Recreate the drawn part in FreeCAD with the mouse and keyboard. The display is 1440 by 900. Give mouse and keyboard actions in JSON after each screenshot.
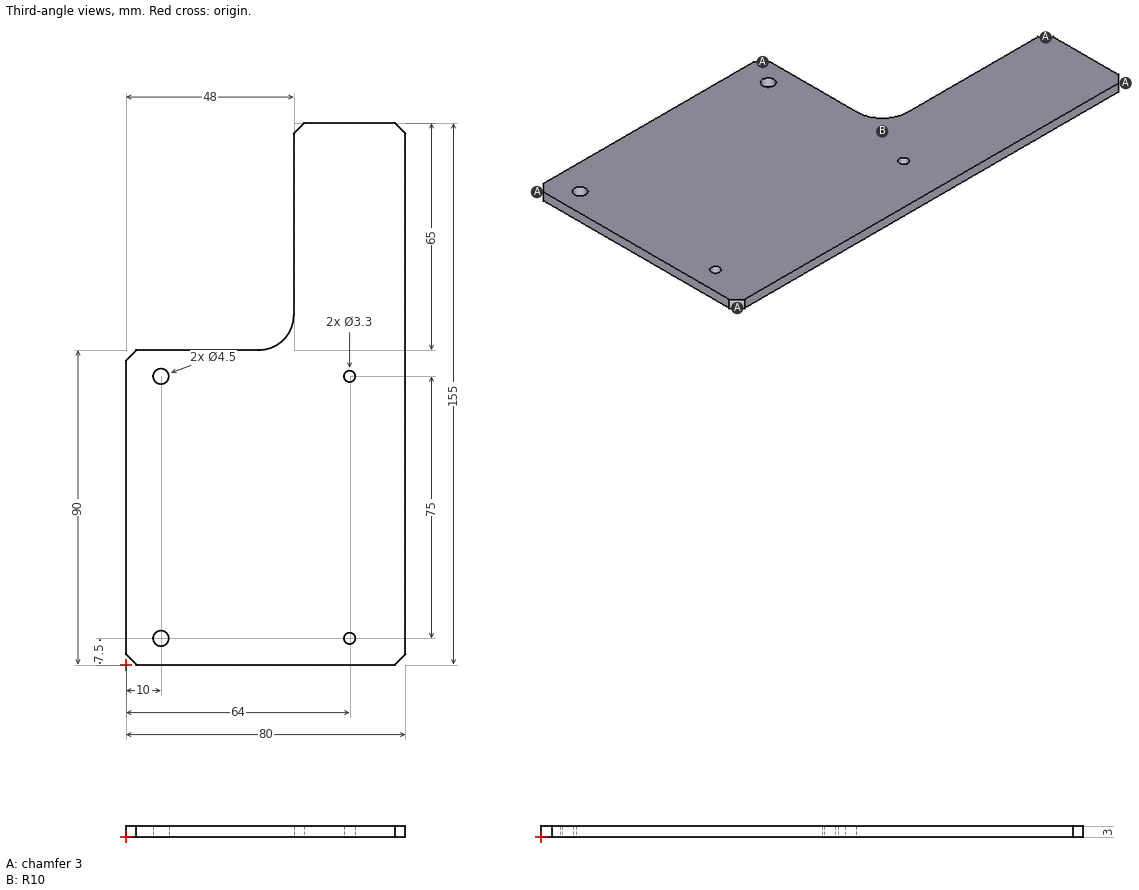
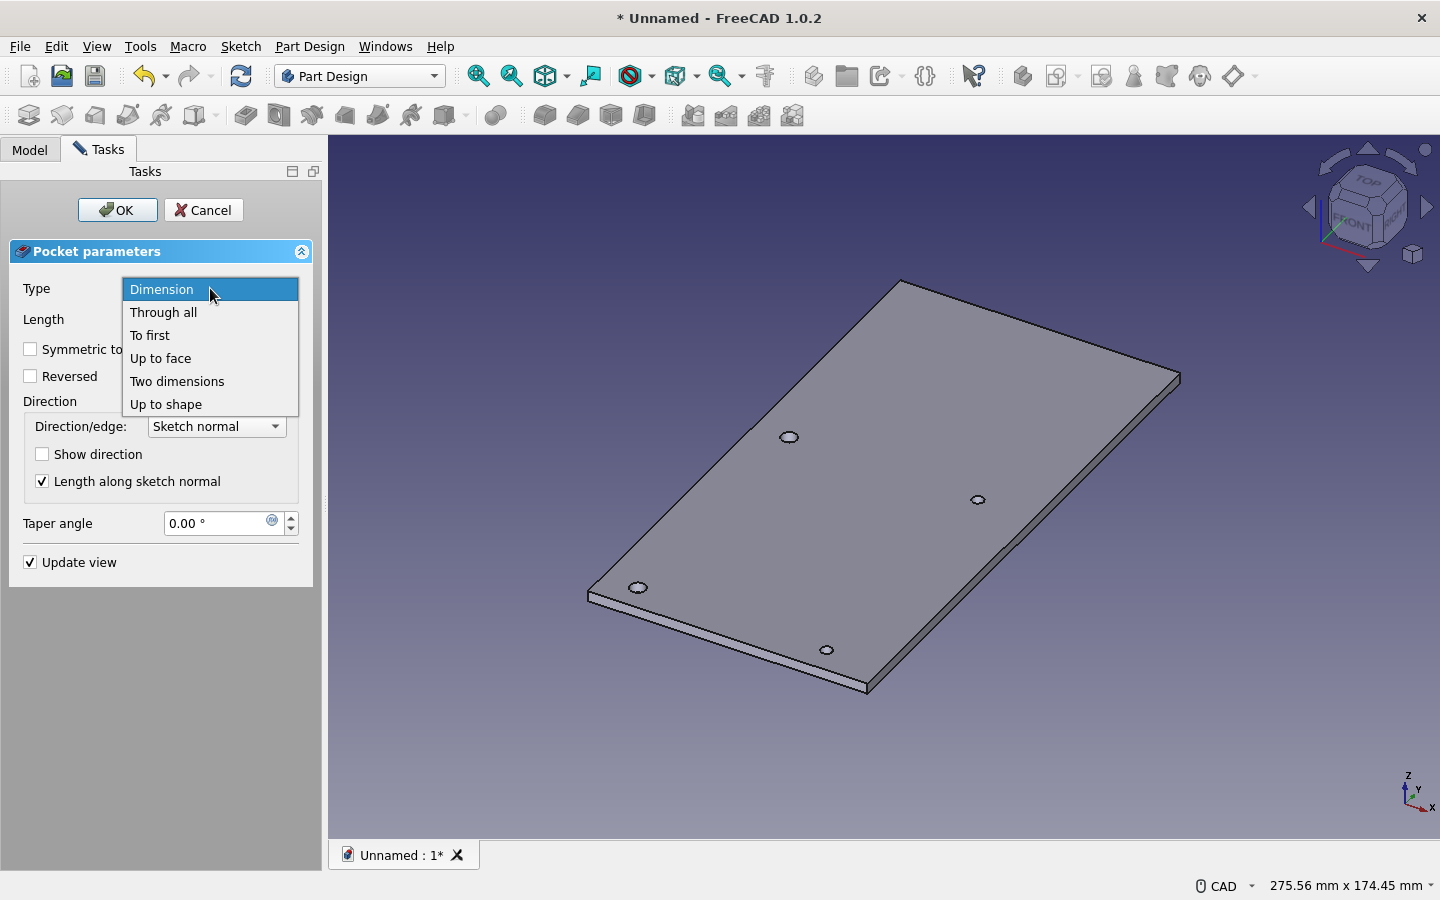
{"action": "left_click", "coordinate": [208, 312]}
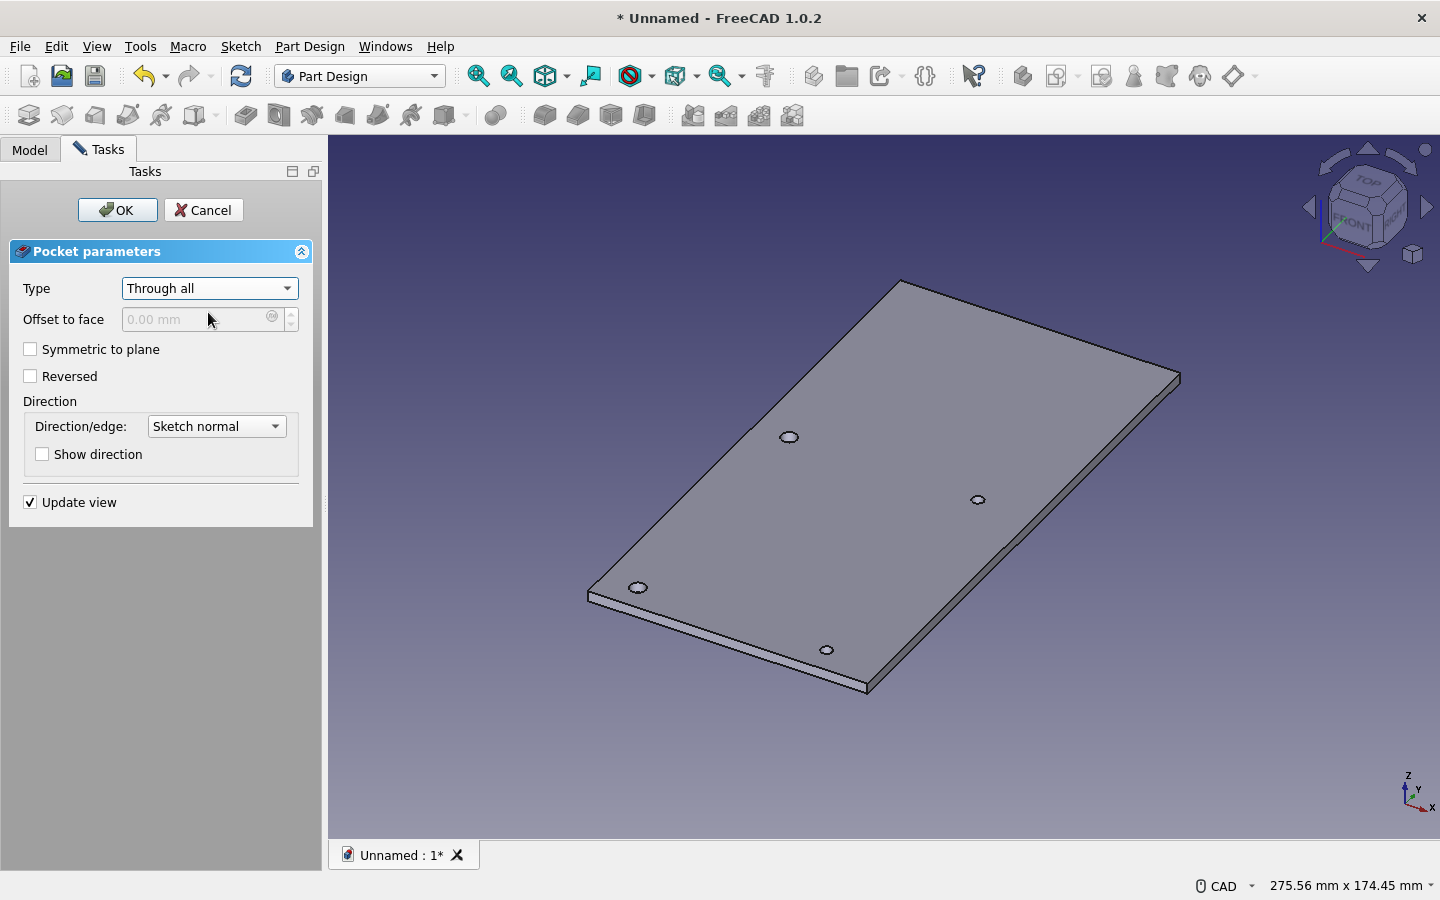
{"action": "left_click", "coordinate": [118, 210]}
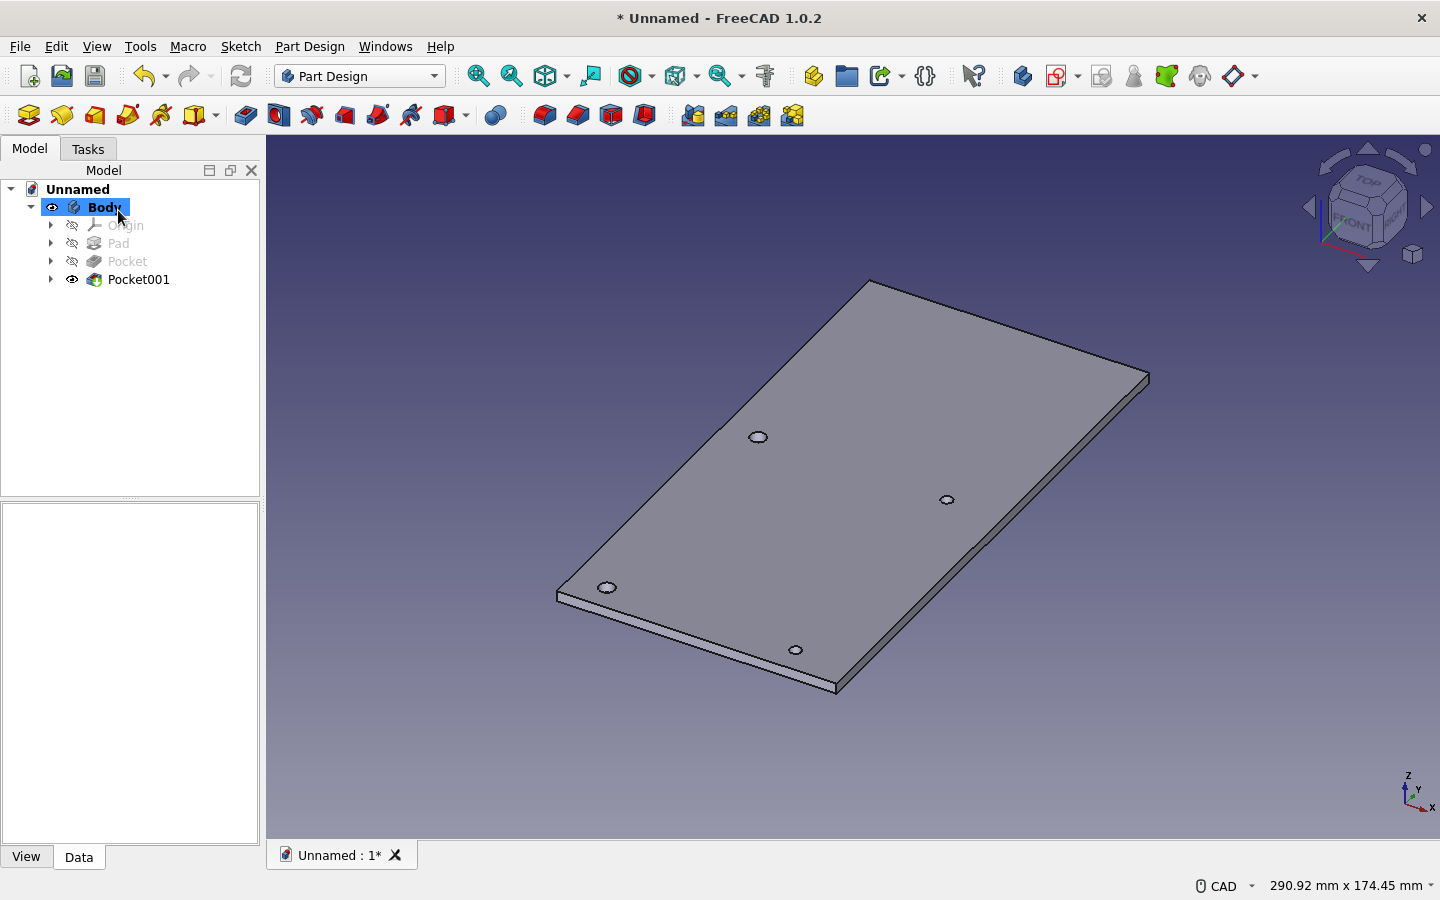
{"action": "left_click", "coordinate": [808, 525]}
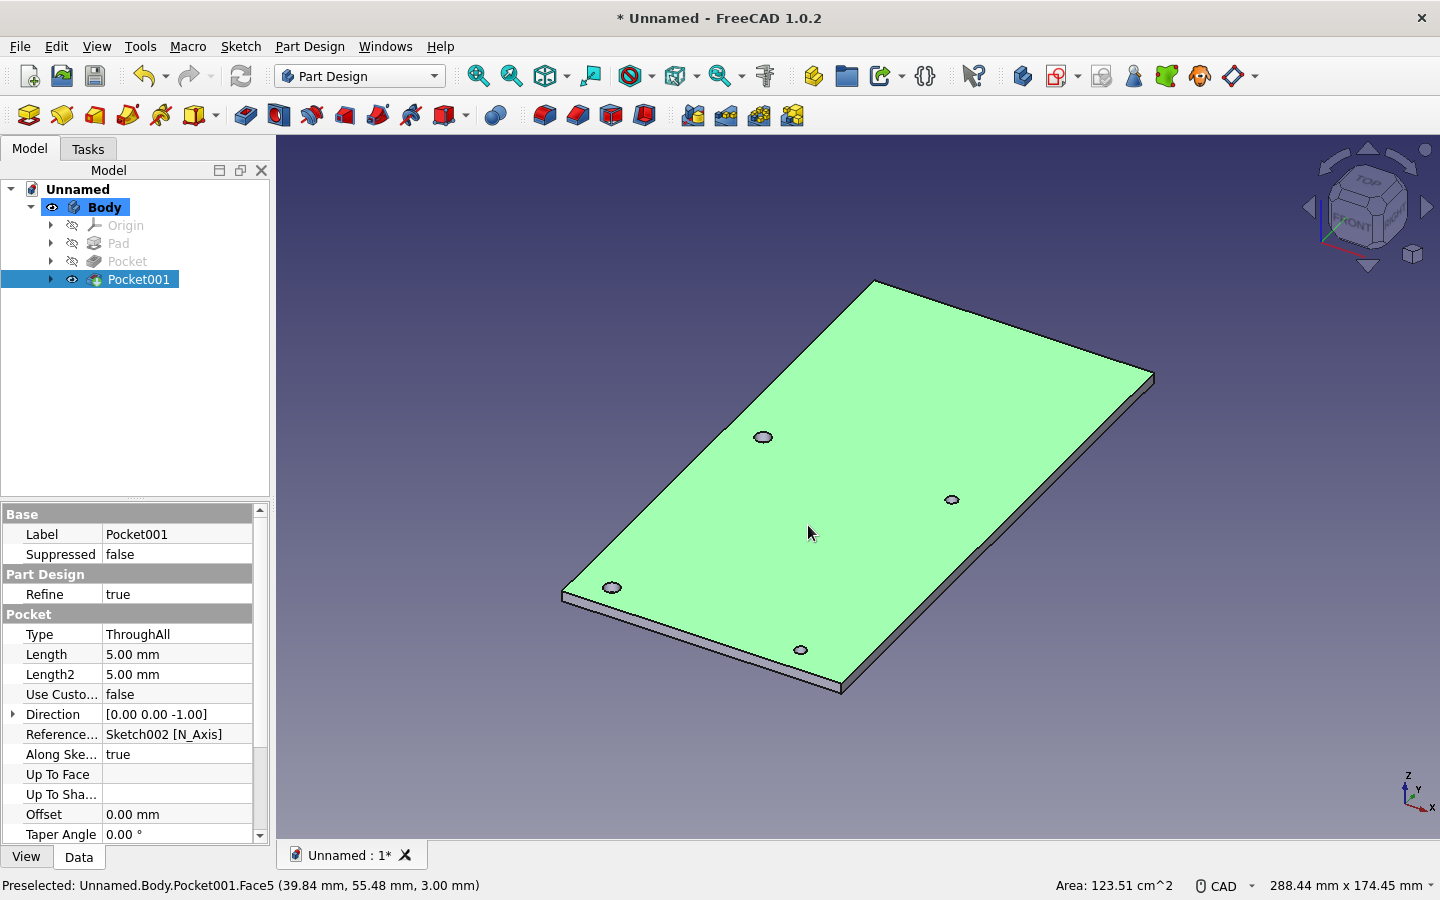
{"action": "left_click", "coordinate": [1056, 76]}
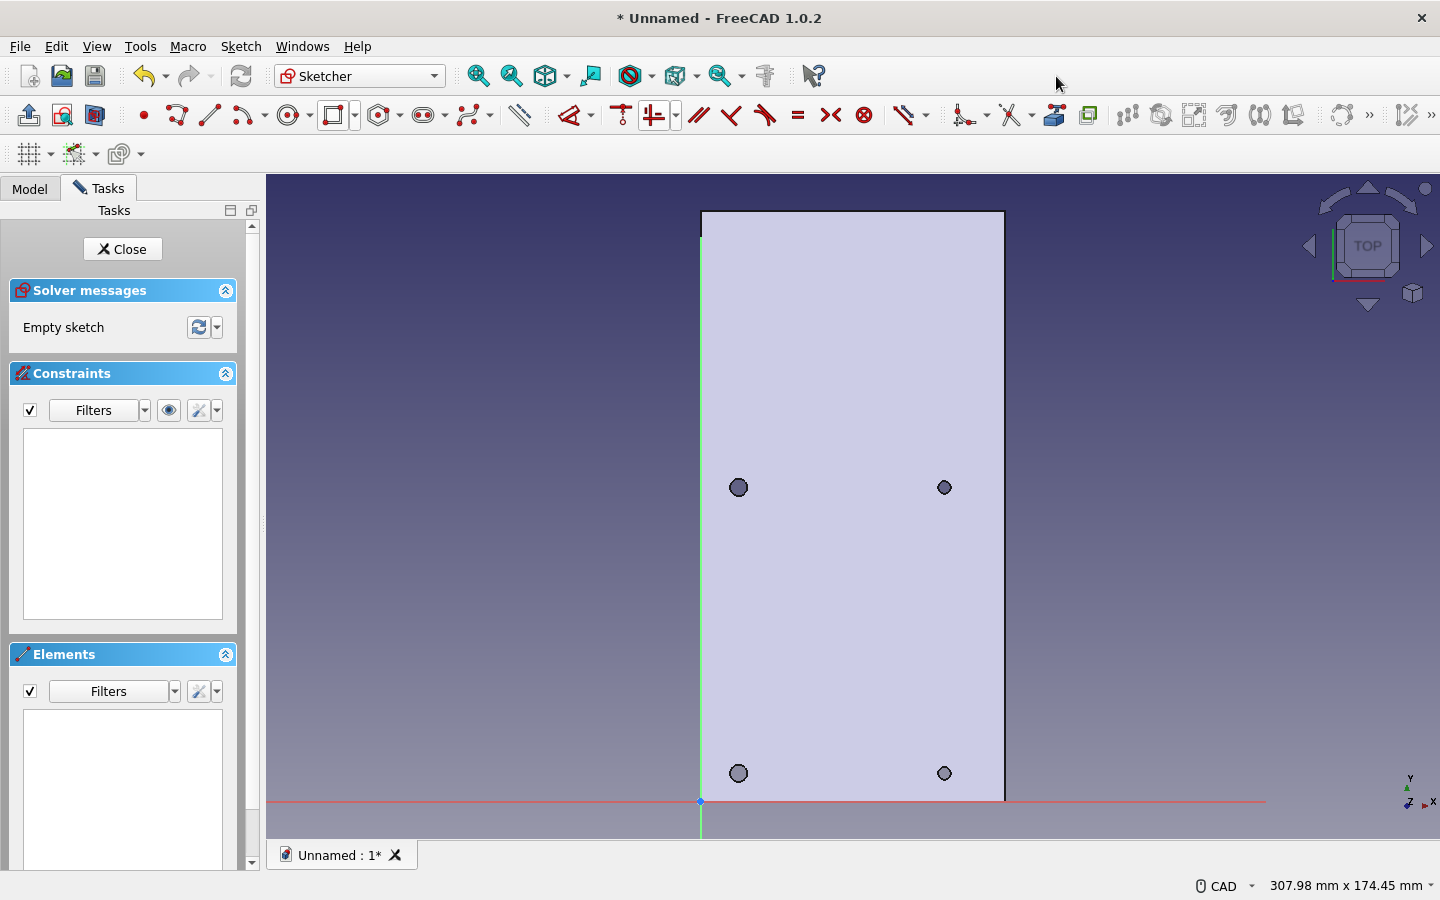
{"action": "scroll", "coordinate": [769, 507], "scroll_direction": "down", "scroll_amount": 2}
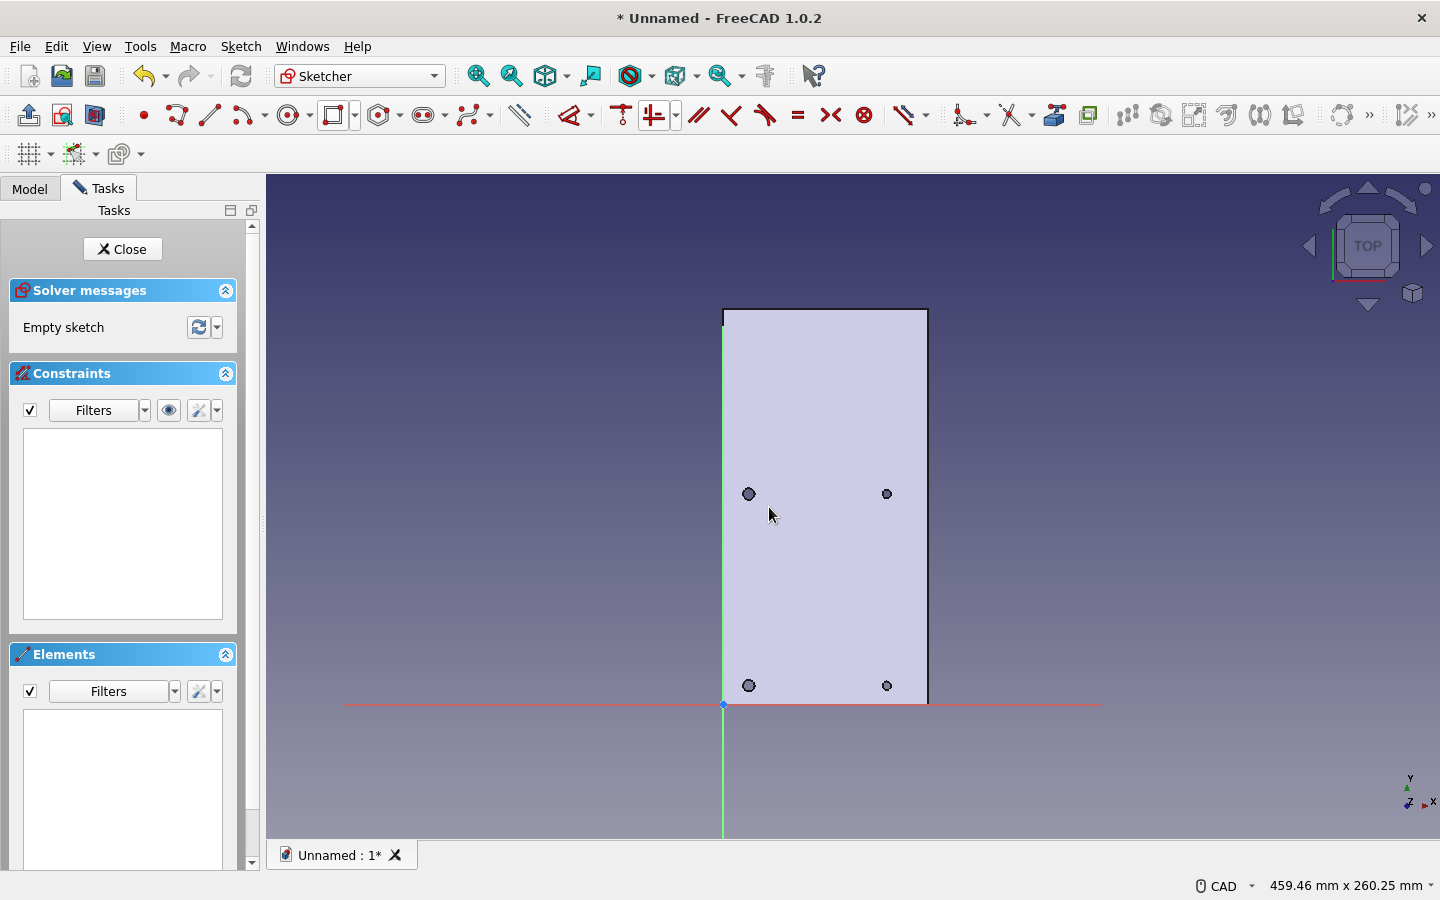
{"action": "key", "text": "g r"}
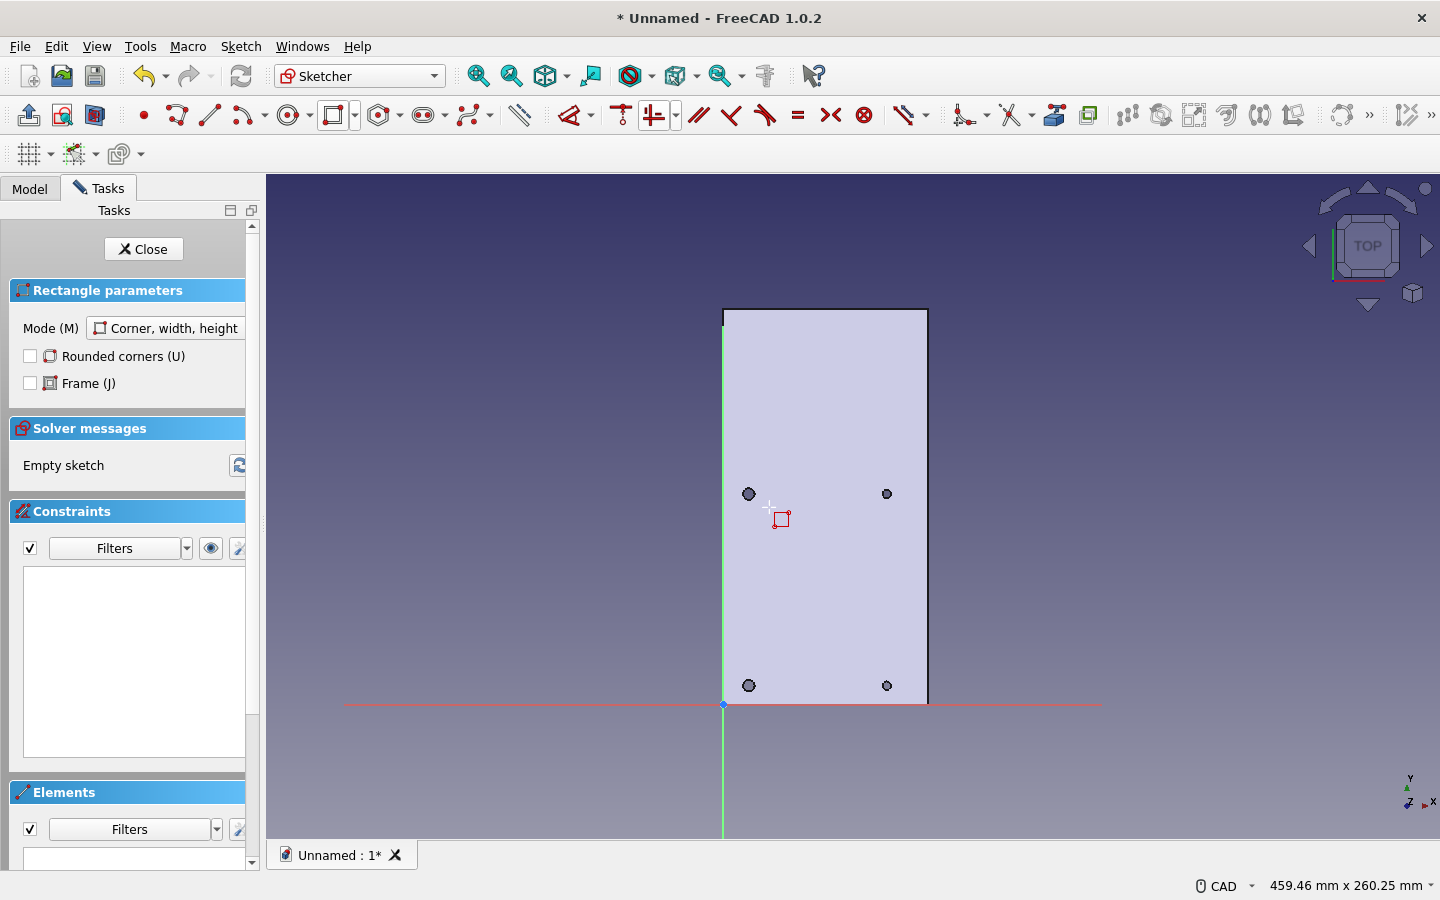
{"action": "left_click", "coordinate": [723, 309]}
{"action": "mouse_move", "coordinate": [846, 475]}